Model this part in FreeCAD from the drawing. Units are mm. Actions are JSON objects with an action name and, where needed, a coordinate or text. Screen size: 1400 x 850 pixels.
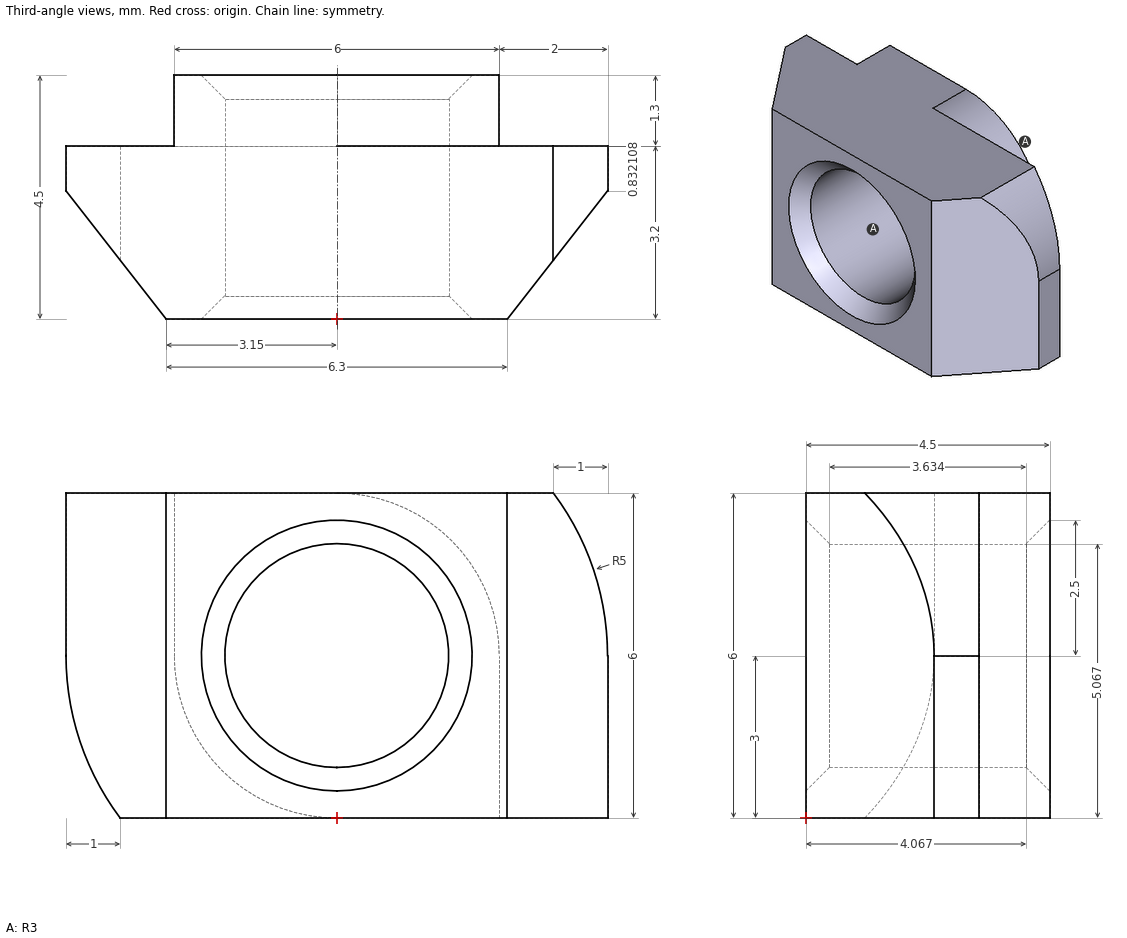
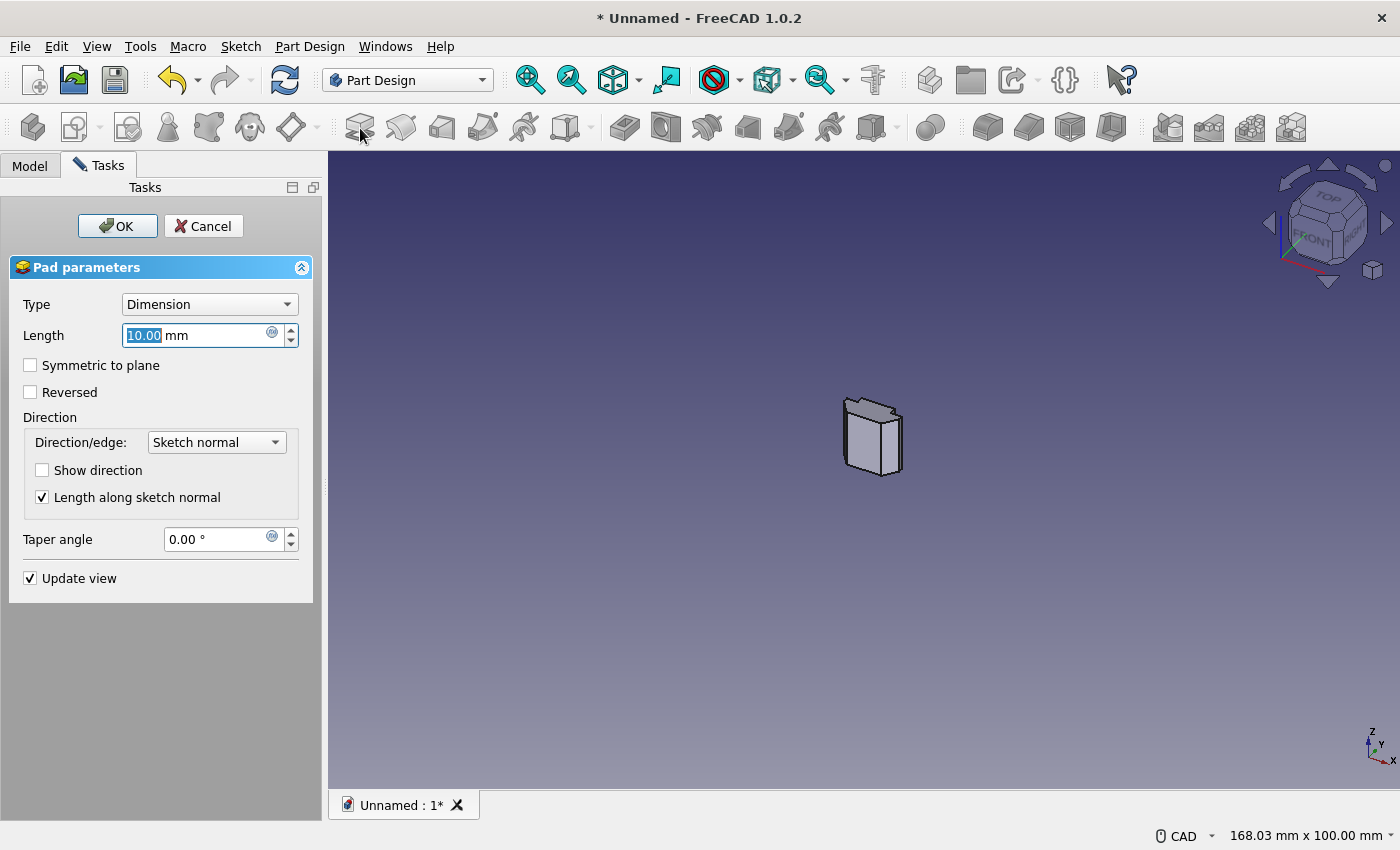
{"action": "type", "text": "6"}
{"action": "key", "text": "Tab"}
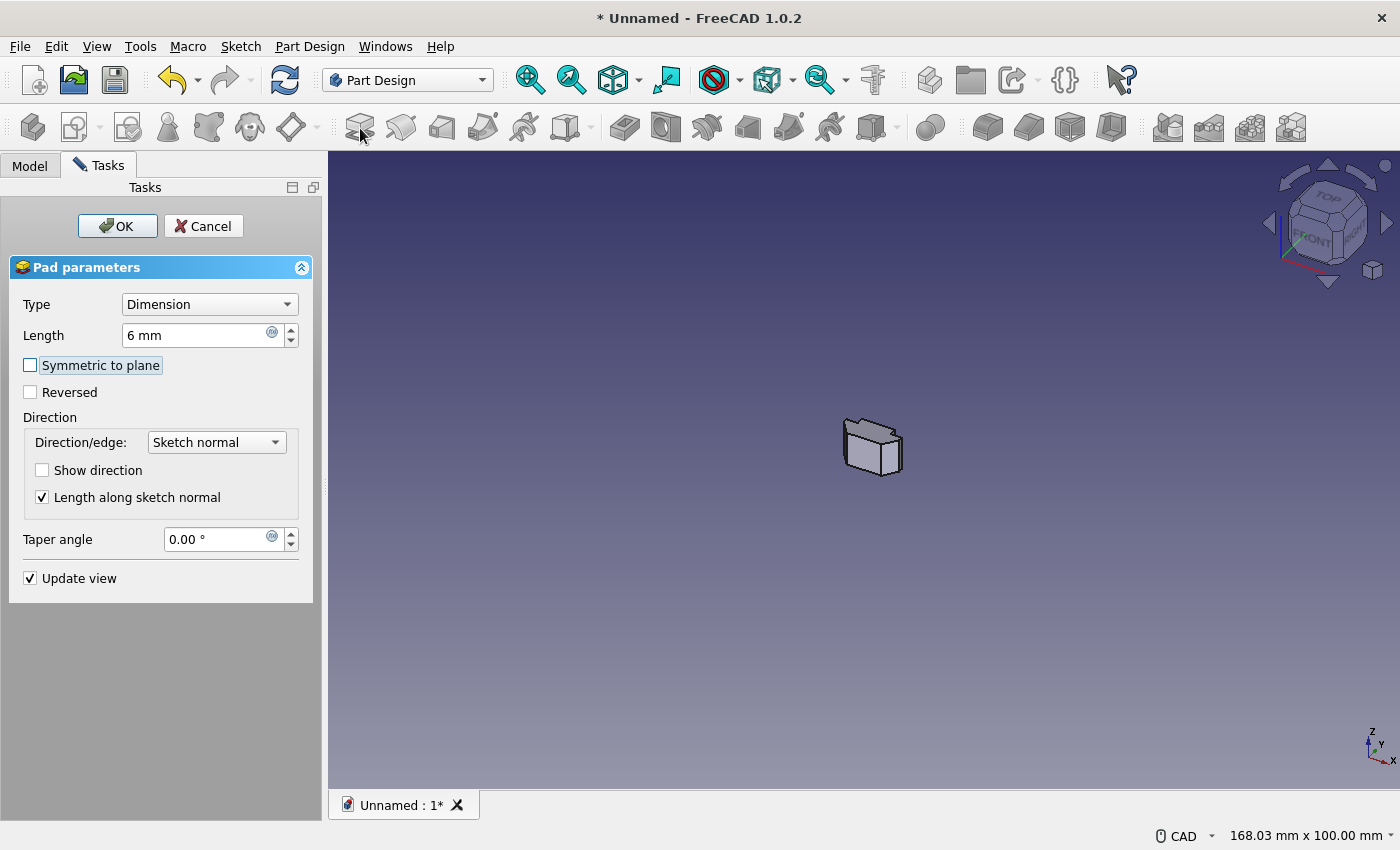
{"action": "left_click", "coordinate": [118, 226]}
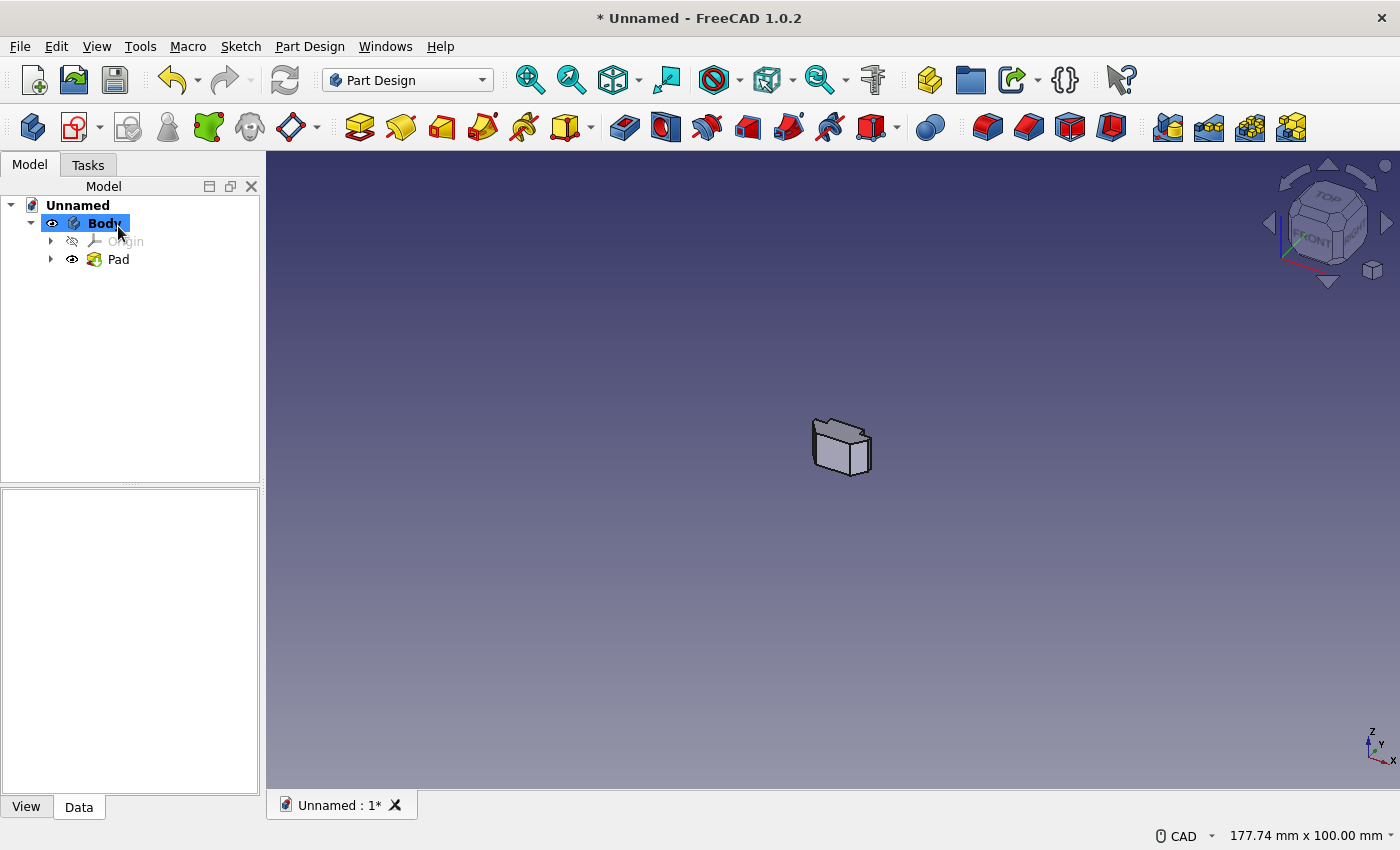
{"action": "left_click", "coordinate": [531, 80]}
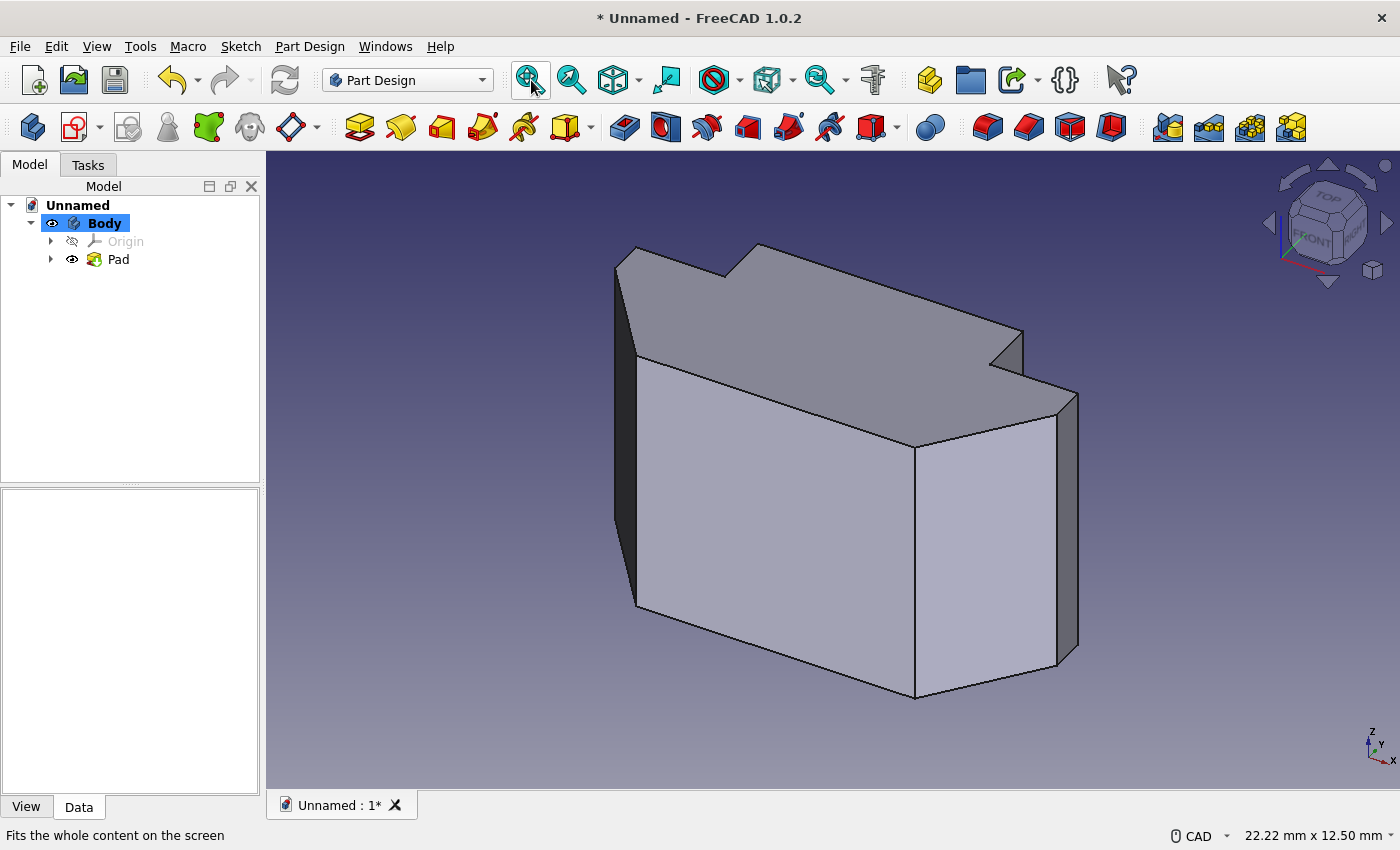
{"action": "left_click", "coordinate": [74, 128]}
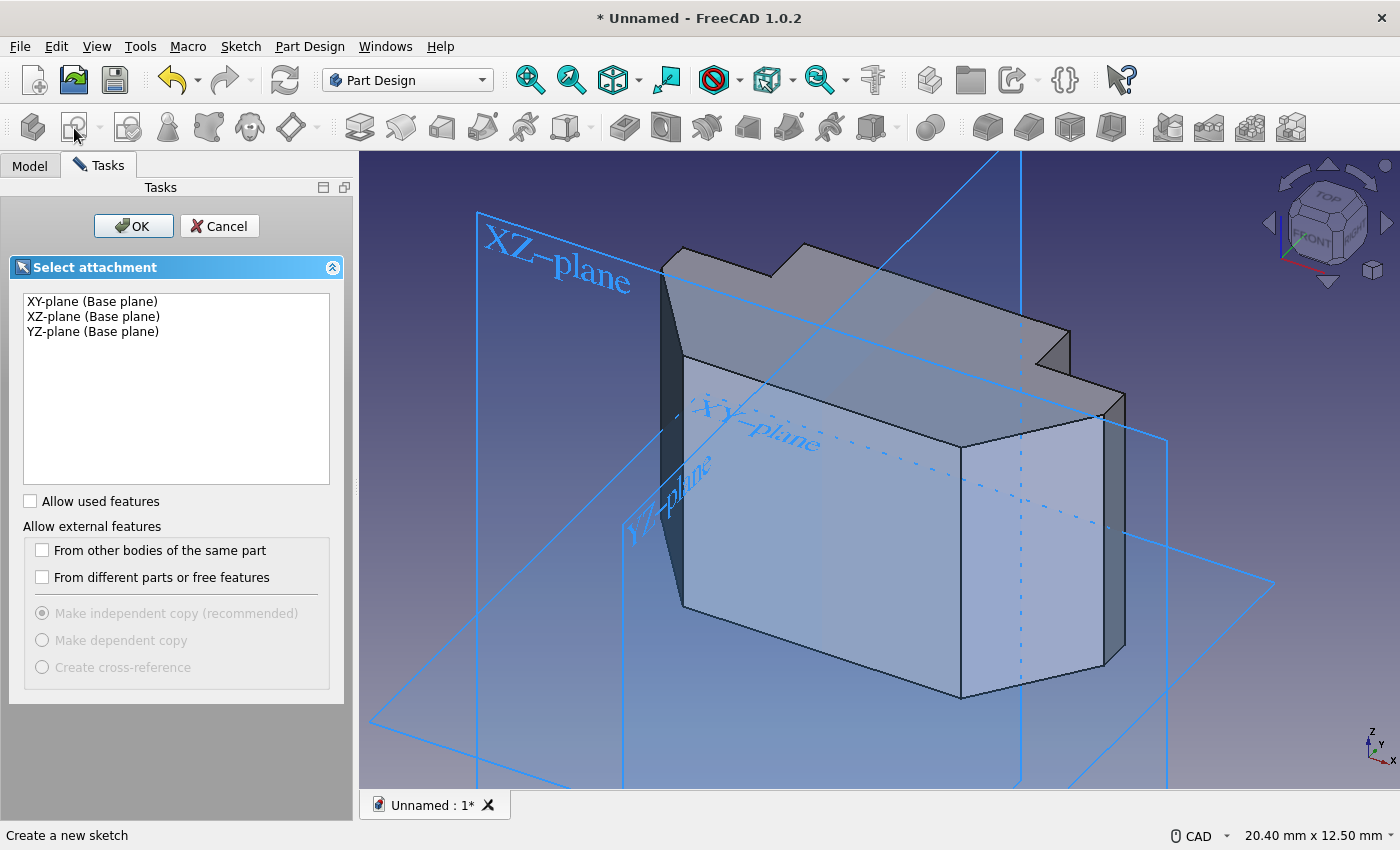
{"action": "left_click", "coordinate": [84, 332]}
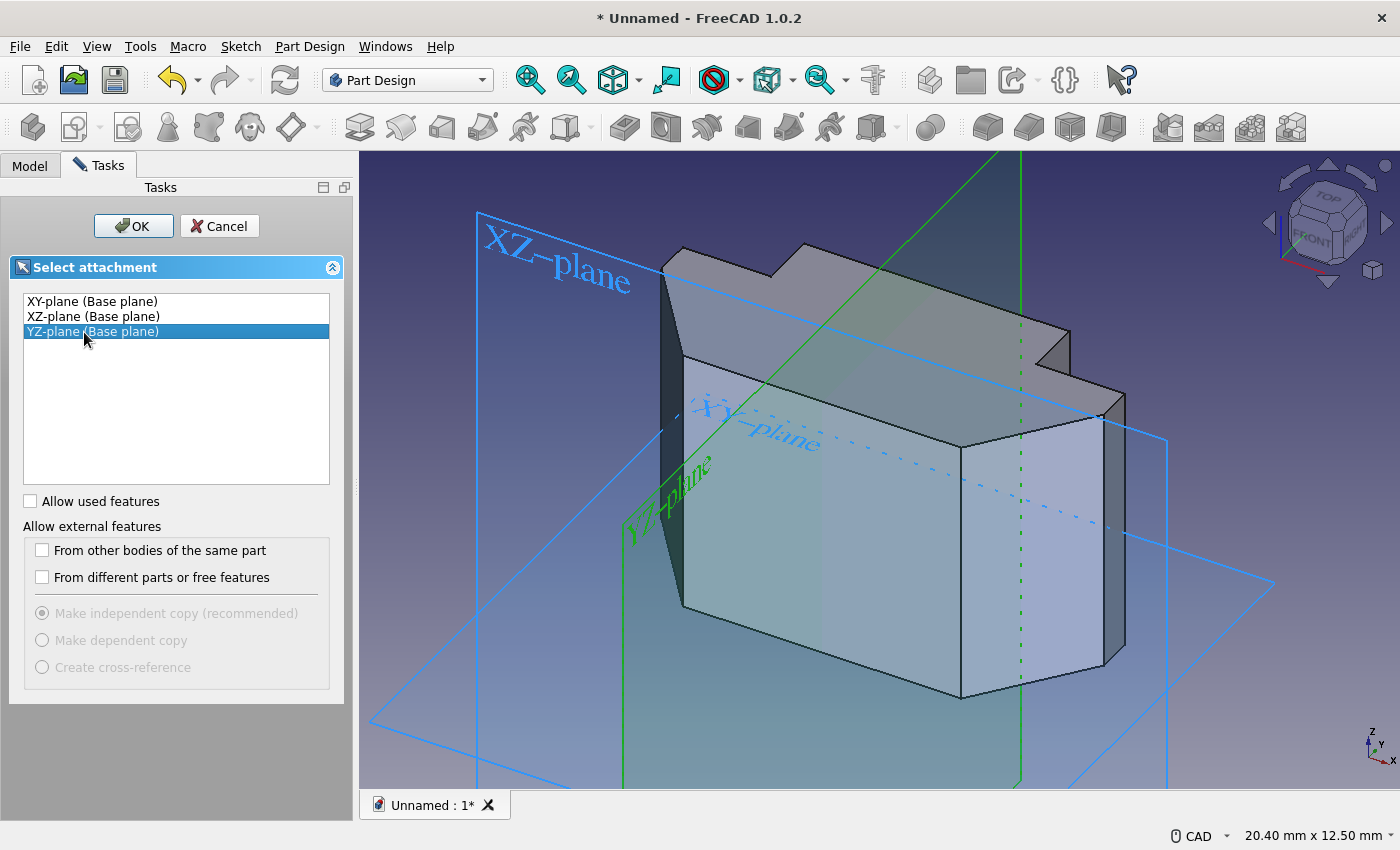
{"action": "left_click", "coordinate": [134, 226]}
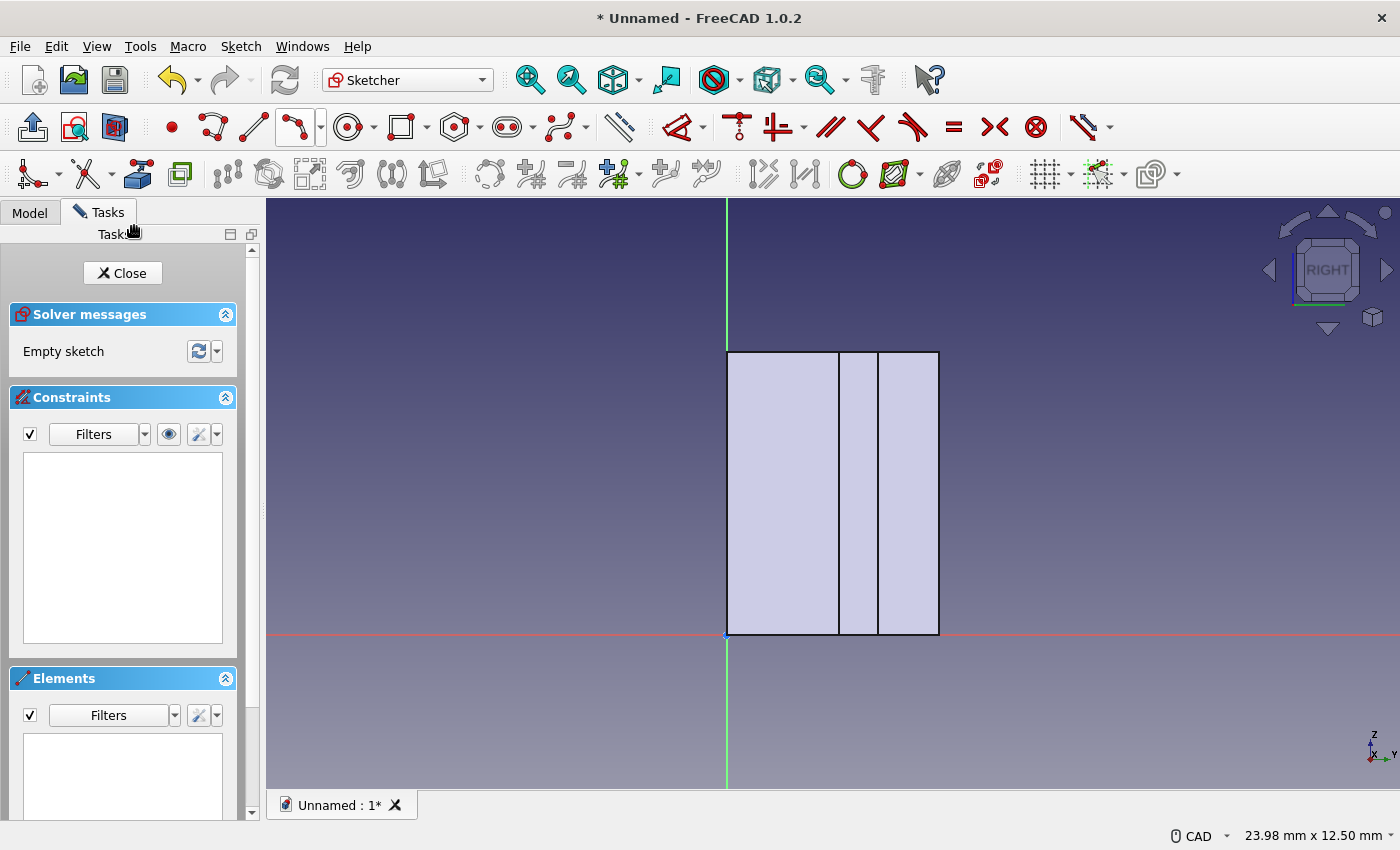
{"action": "left_click", "coordinate": [115, 128]}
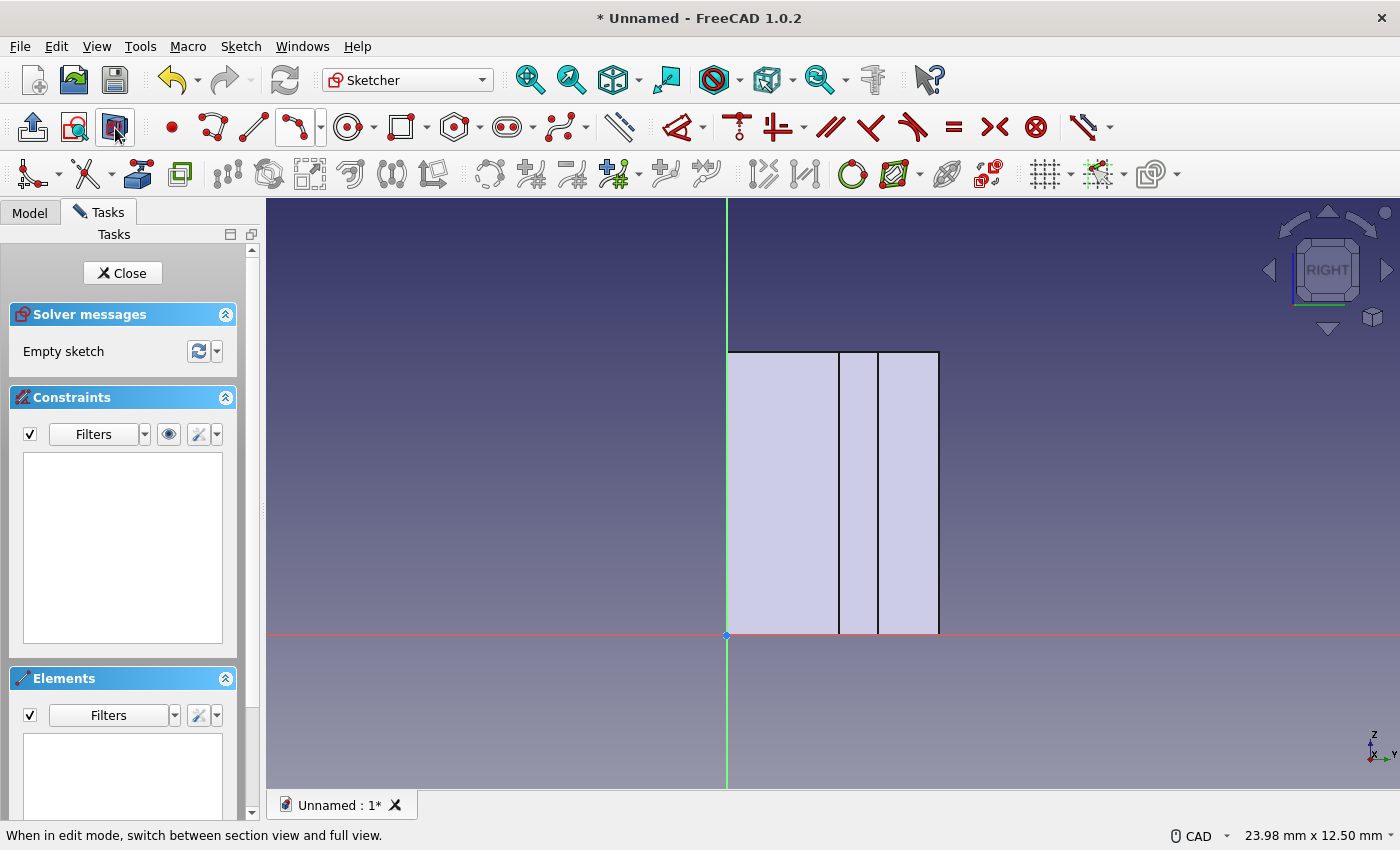
{"action": "scroll", "coordinate": [843, 529], "scroll_direction": "up", "scroll_amount": 2}